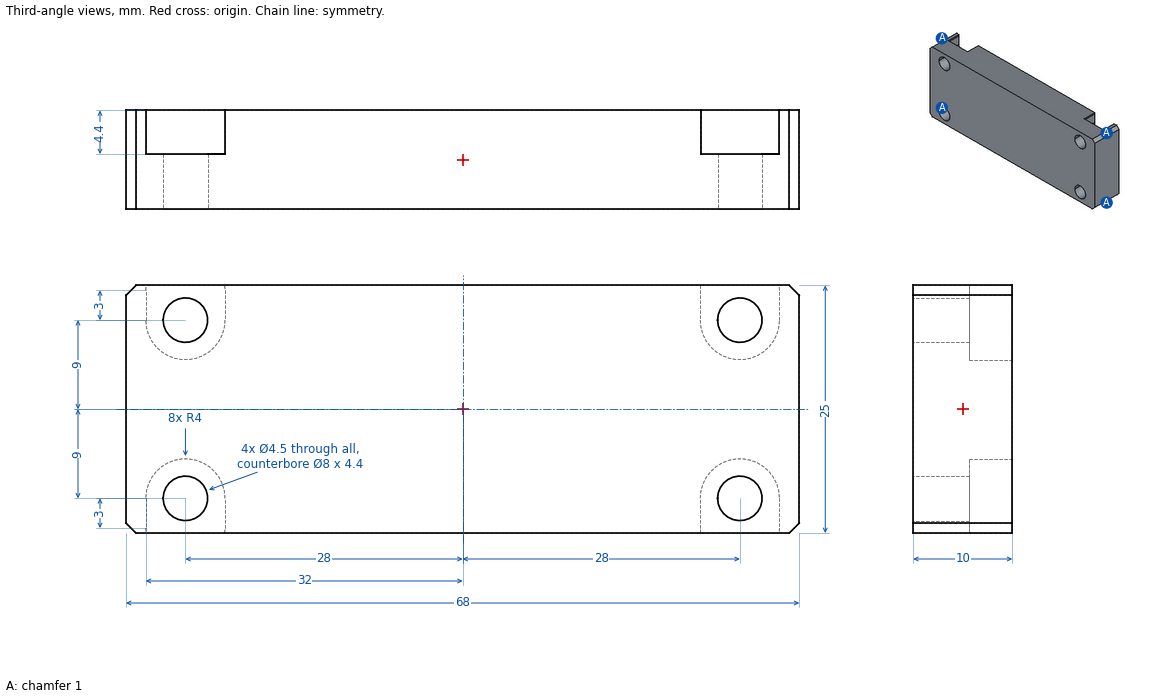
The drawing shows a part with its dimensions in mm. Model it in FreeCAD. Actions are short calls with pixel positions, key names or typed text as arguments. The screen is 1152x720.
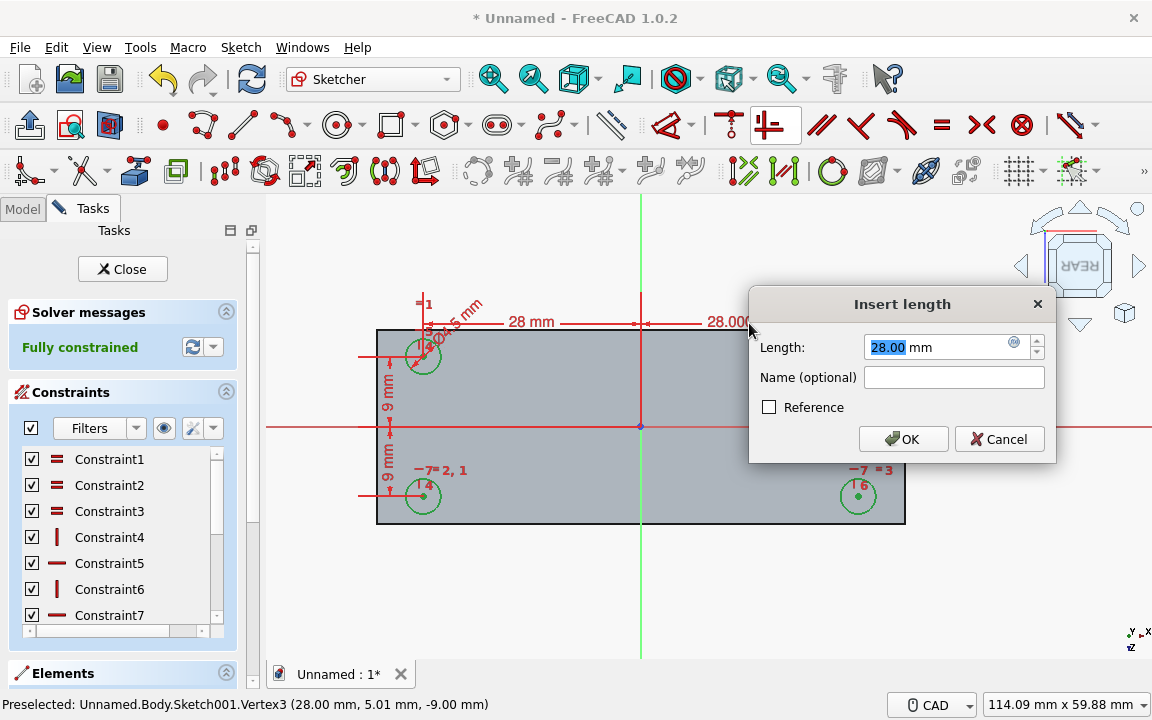
text(28)
key(Return)
key(Escape)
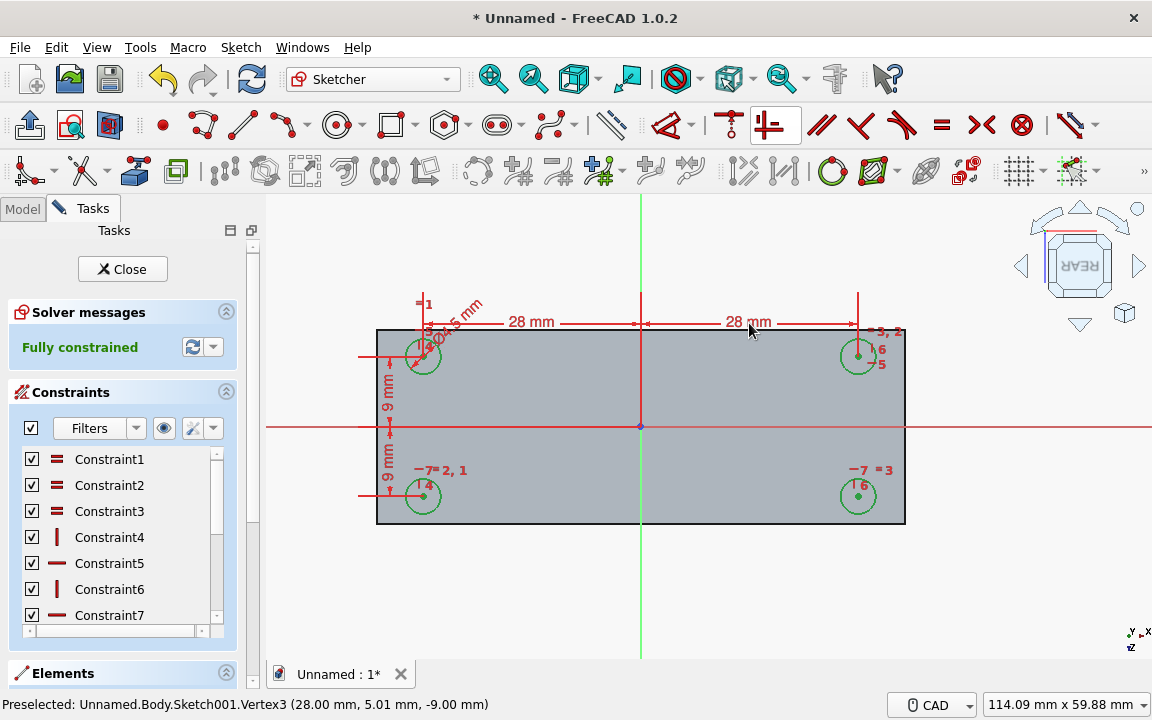
click(123, 269)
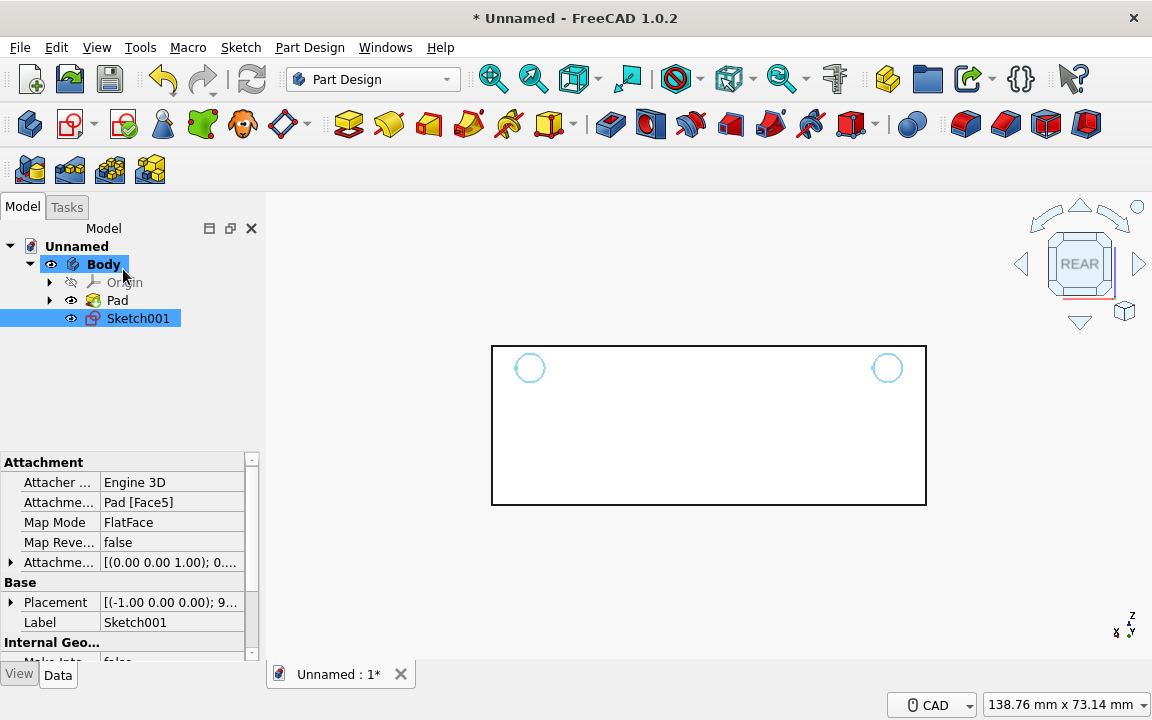
click(652, 124)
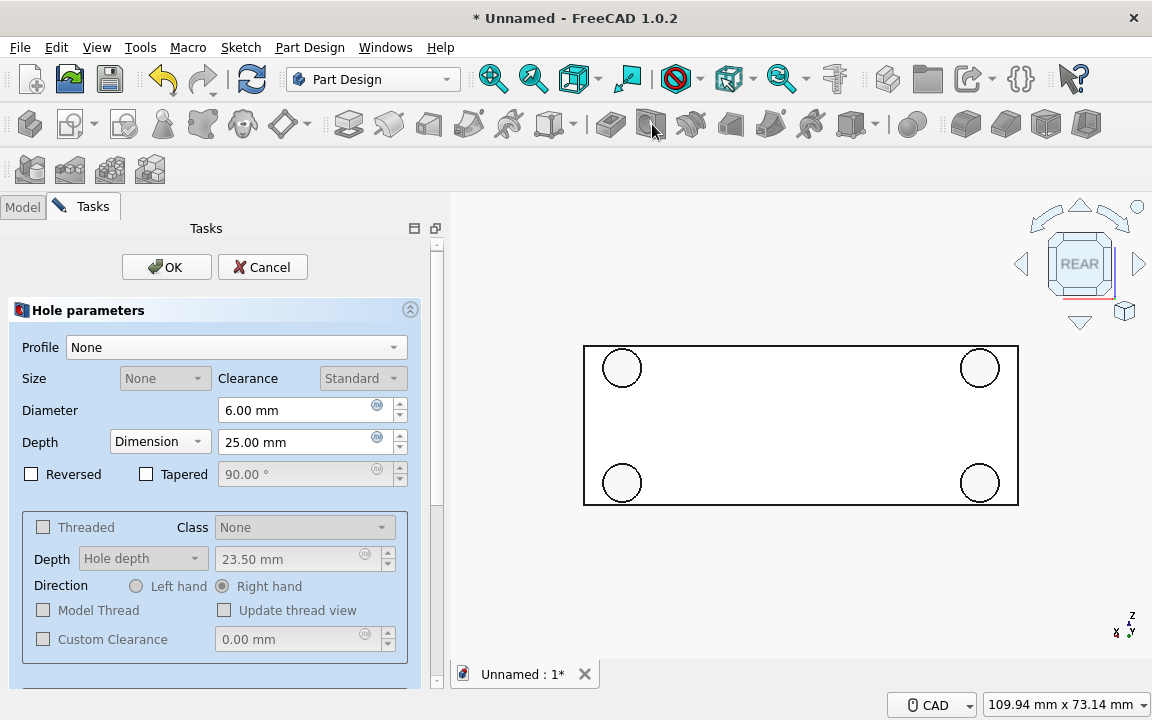
triple_click(305, 410)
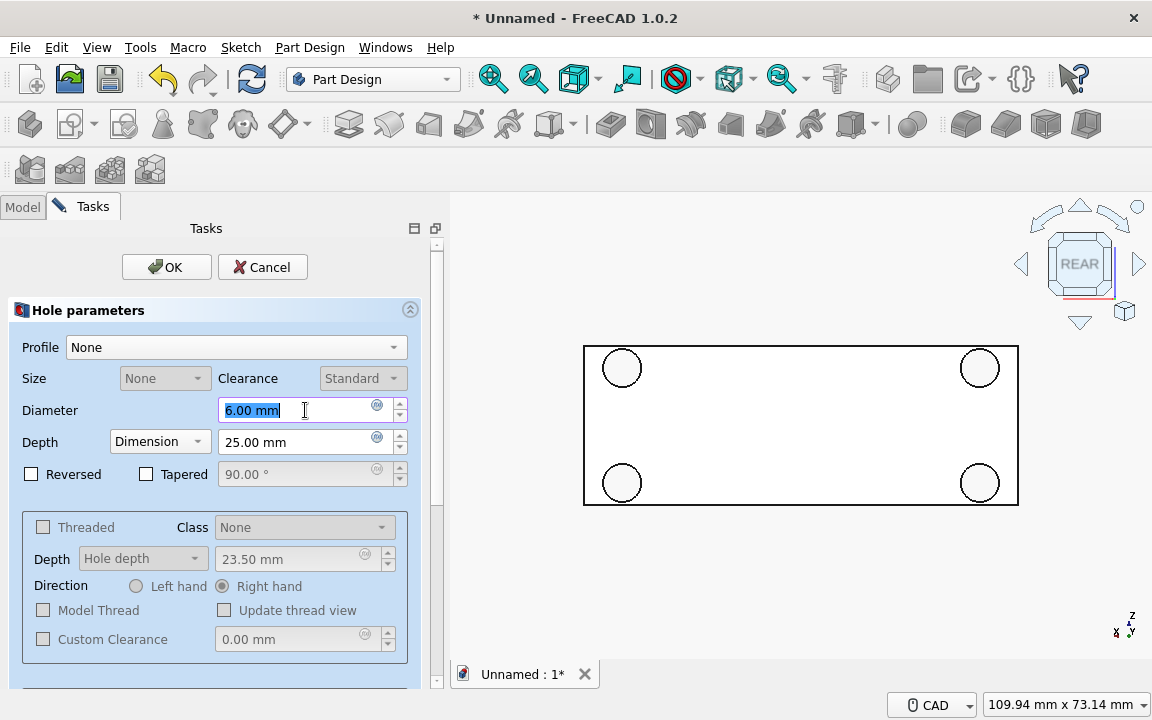
text(4.5)
key(Tab)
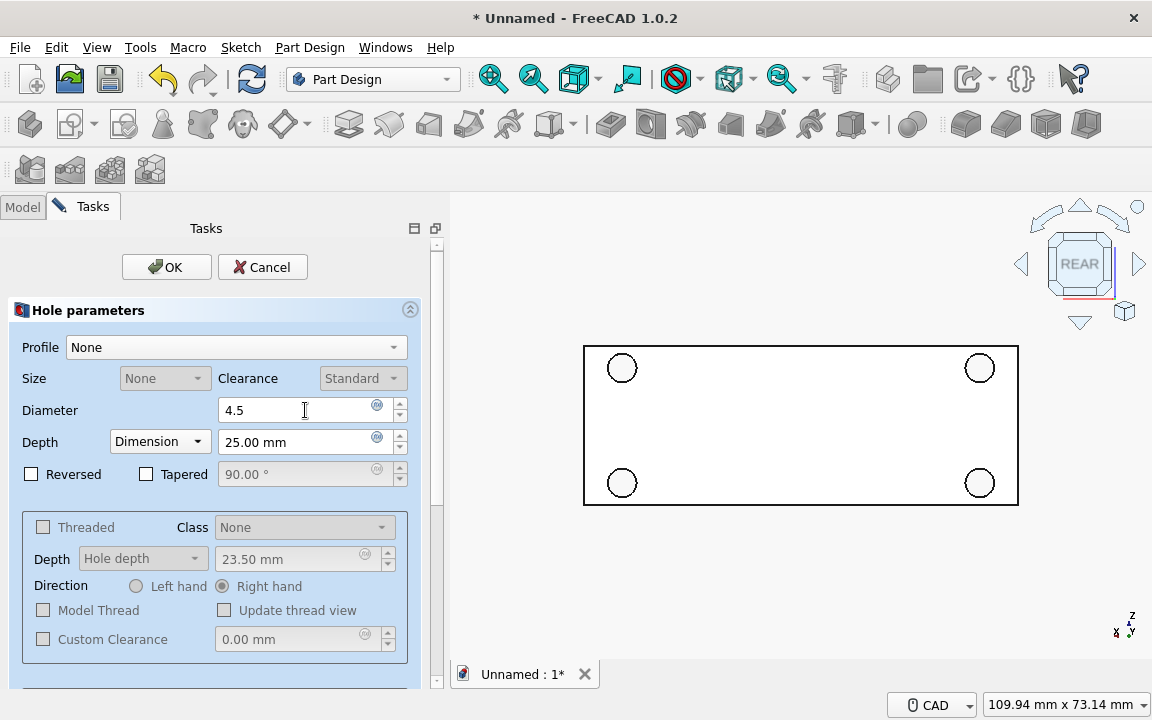
click(161, 442)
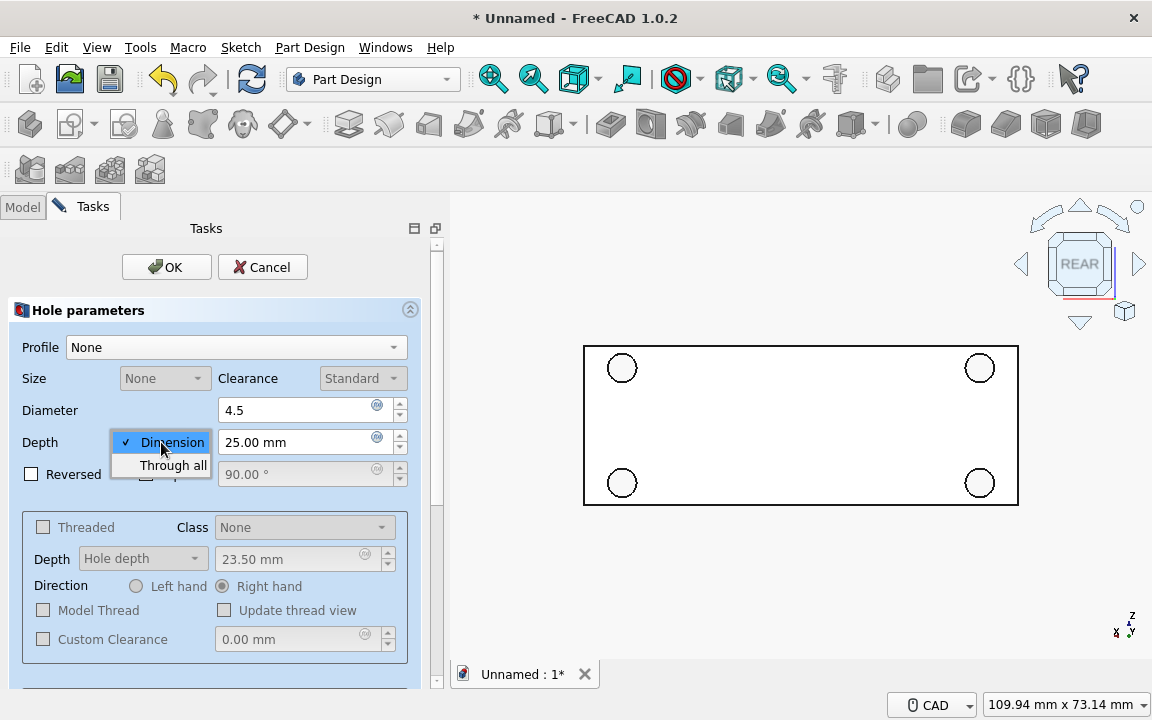
click(160, 466)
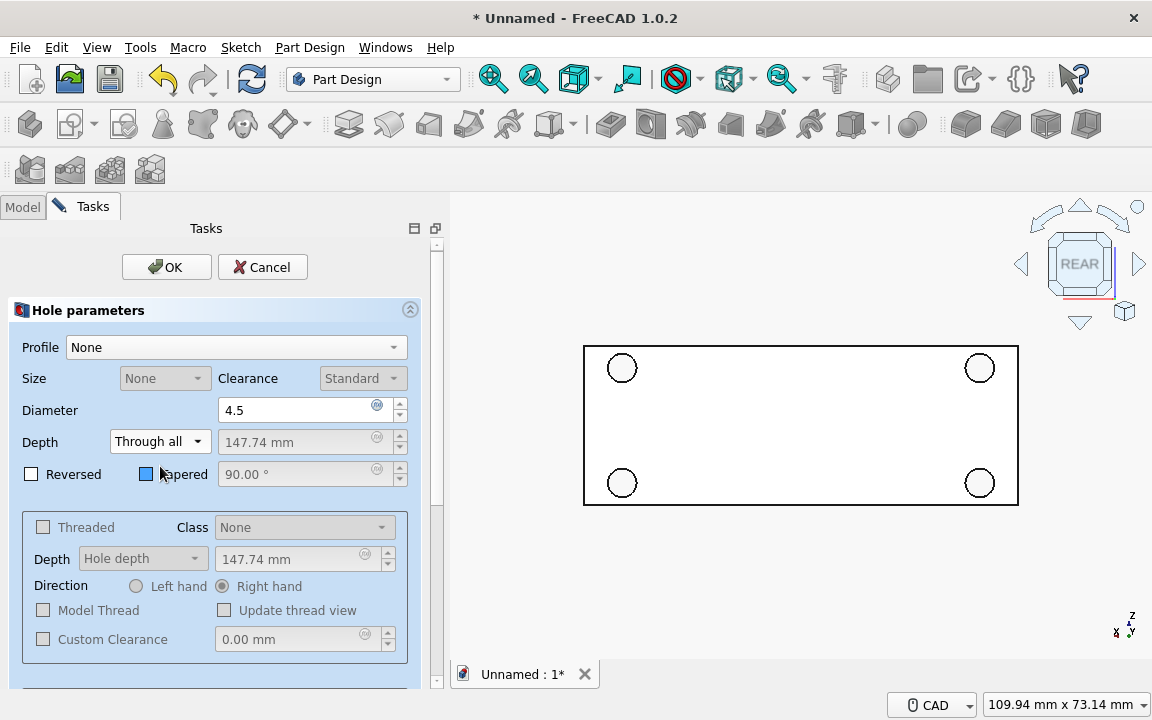
scroll(437, 463, down, 2)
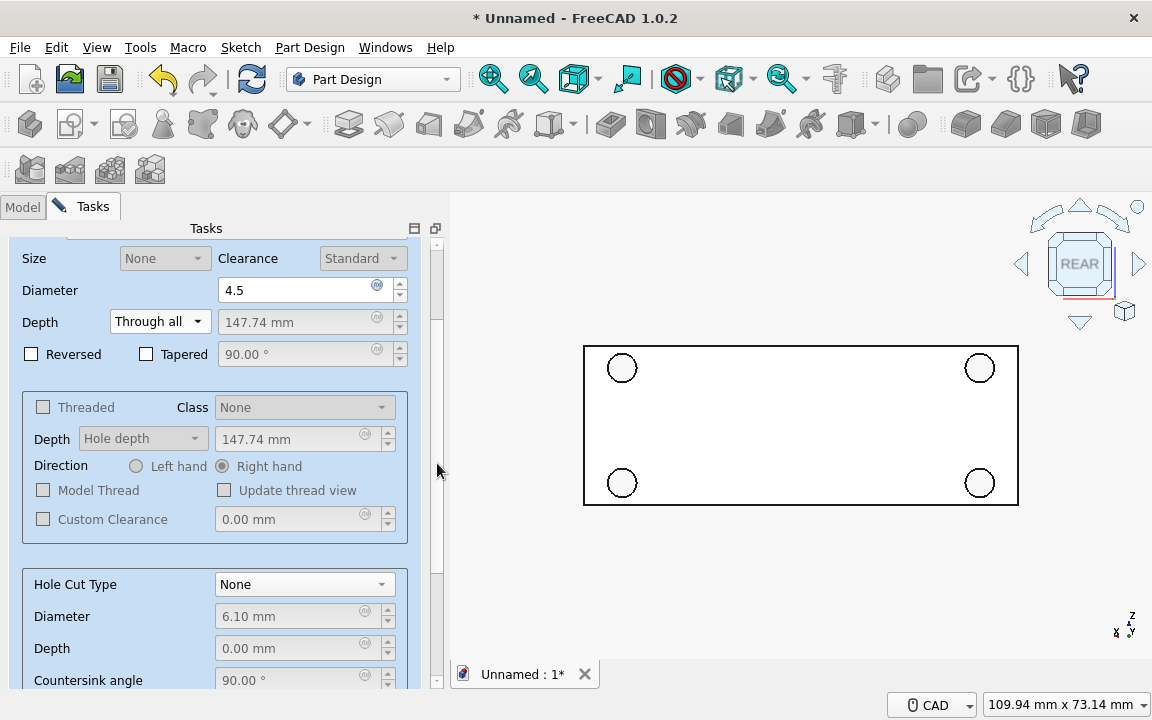
click(306, 584)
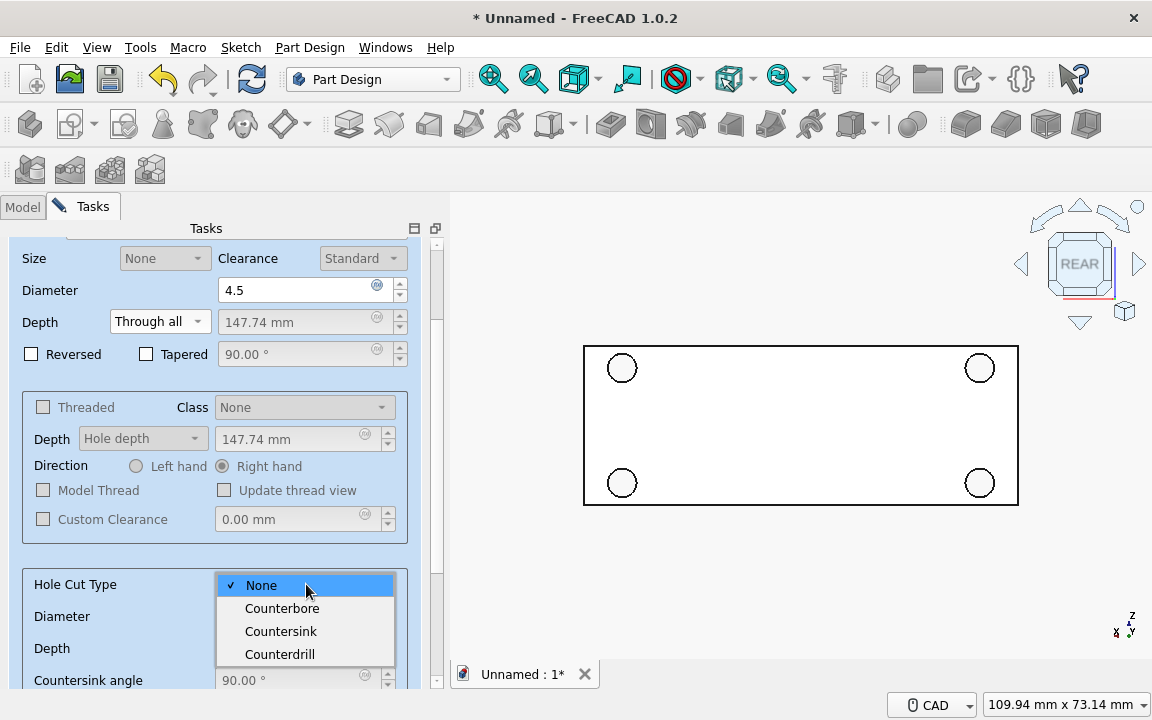
click(304, 608)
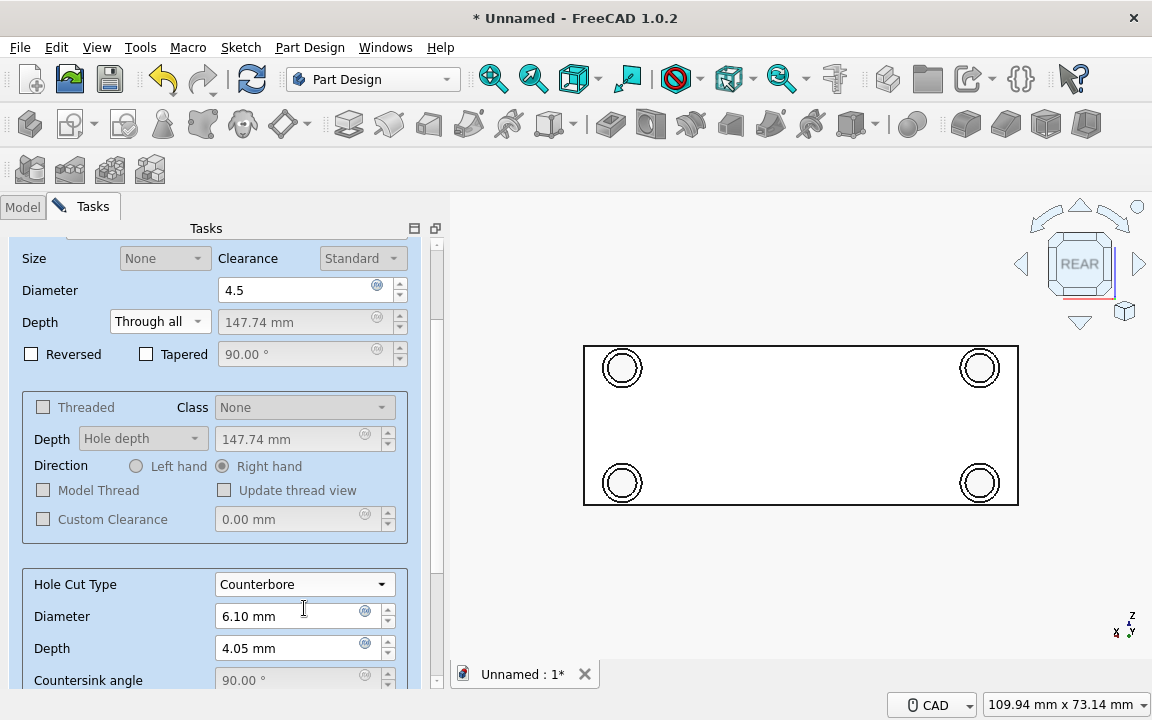
triple_click(298, 616)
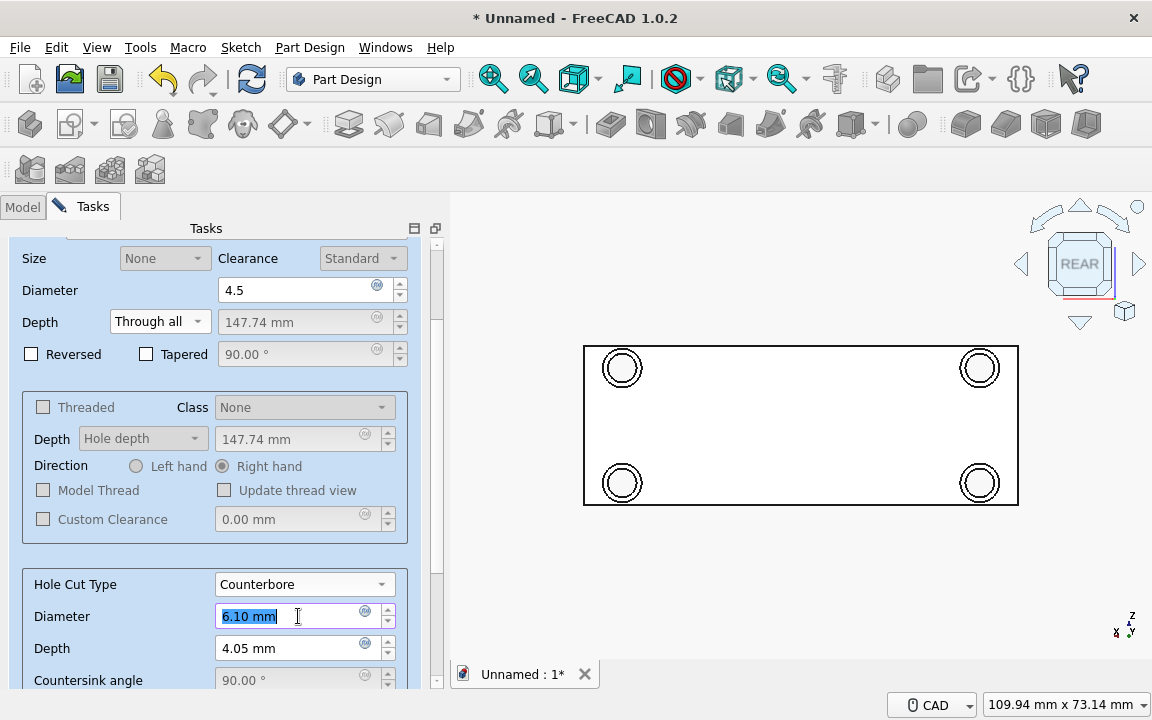
text(8)
key(Tab)